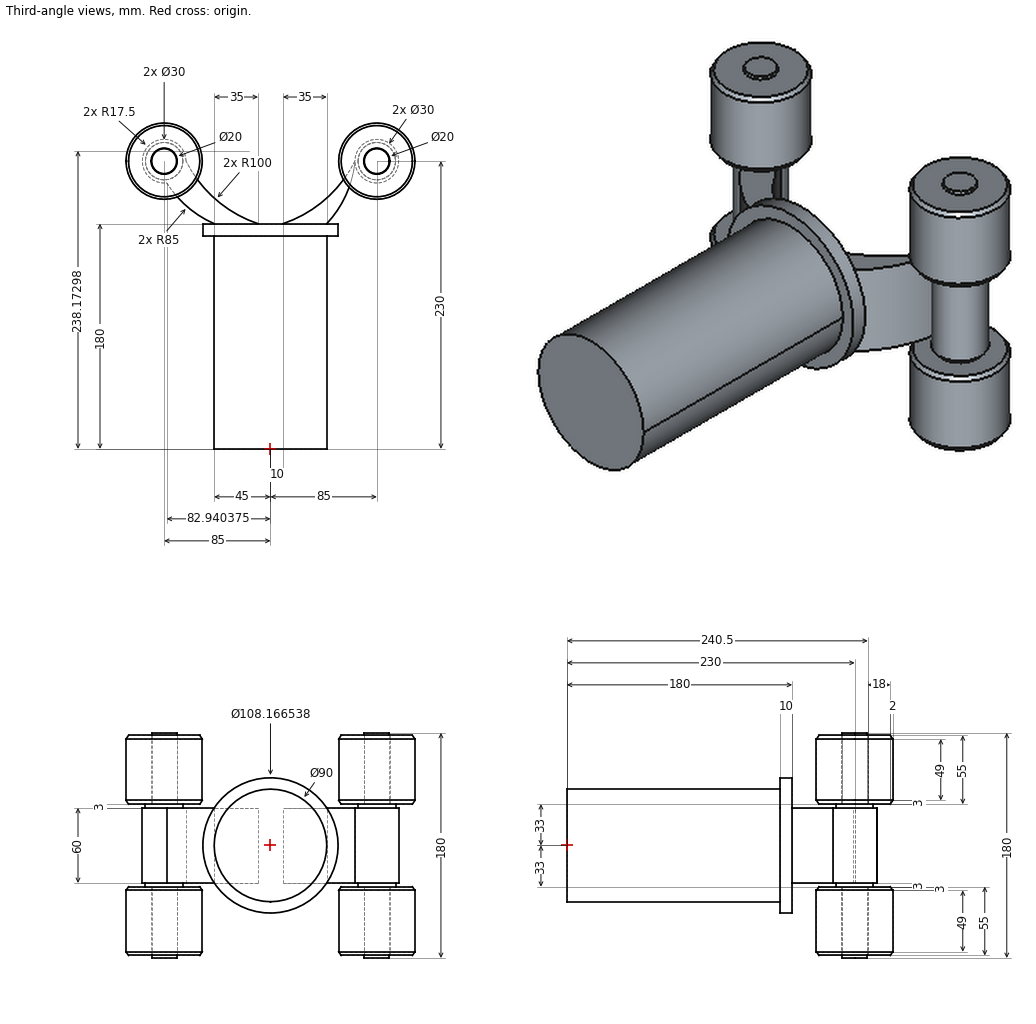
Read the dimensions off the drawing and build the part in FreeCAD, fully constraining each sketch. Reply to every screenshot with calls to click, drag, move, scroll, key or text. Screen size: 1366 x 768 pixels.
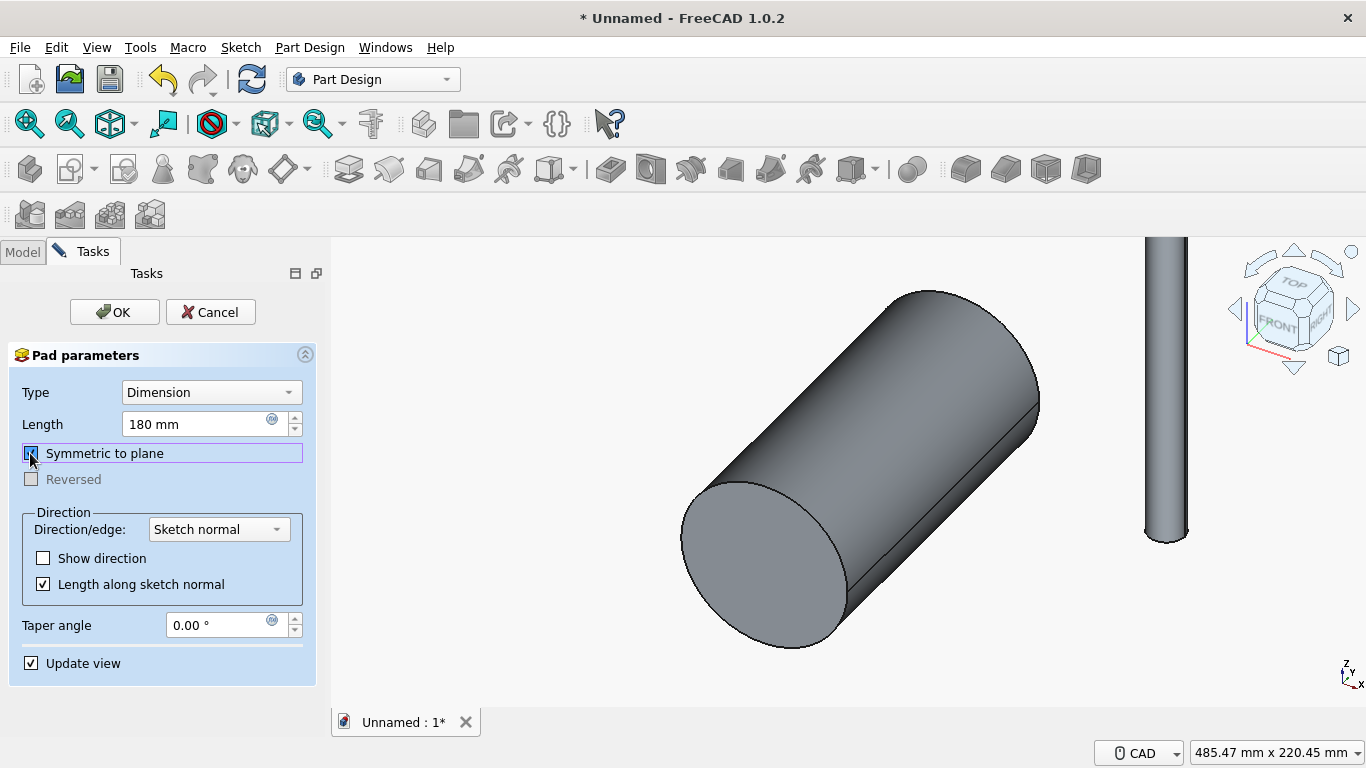
click(115, 312)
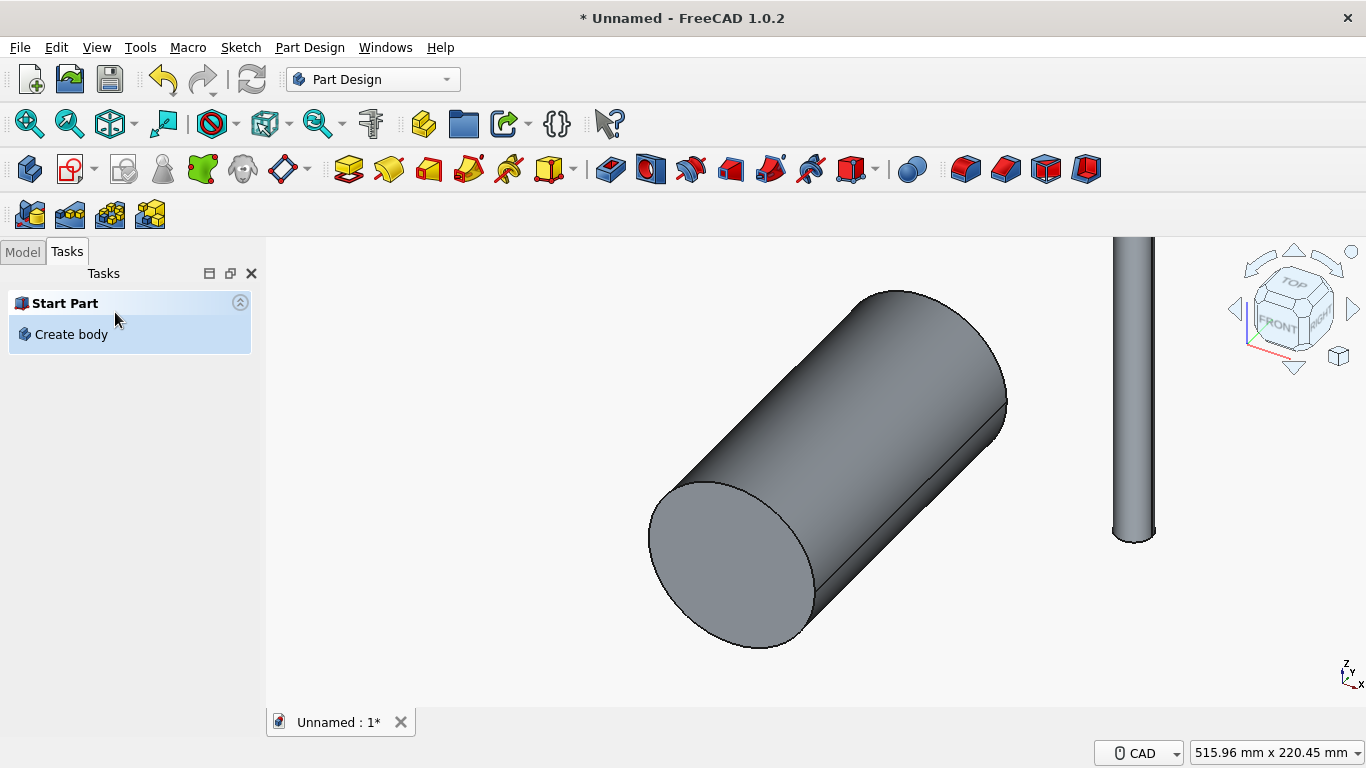
click(30, 124)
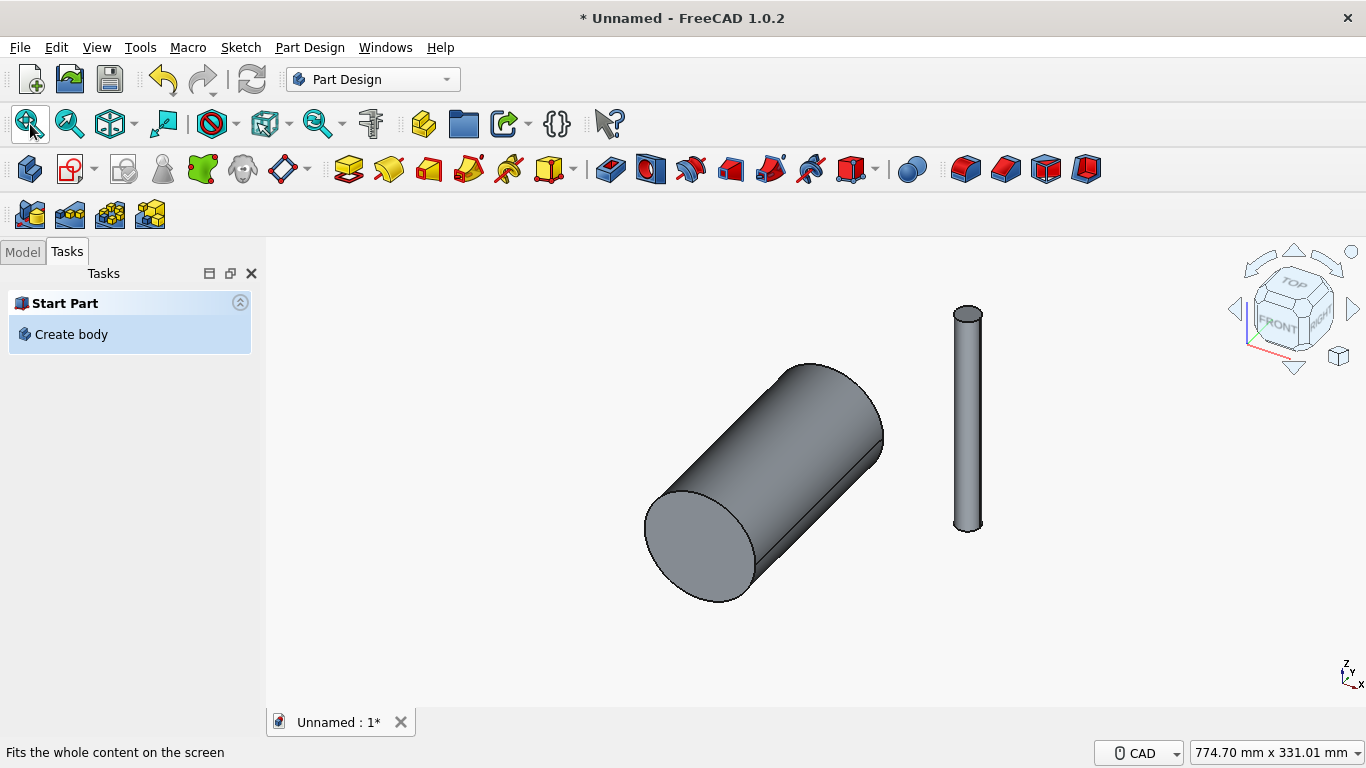
click(30, 170)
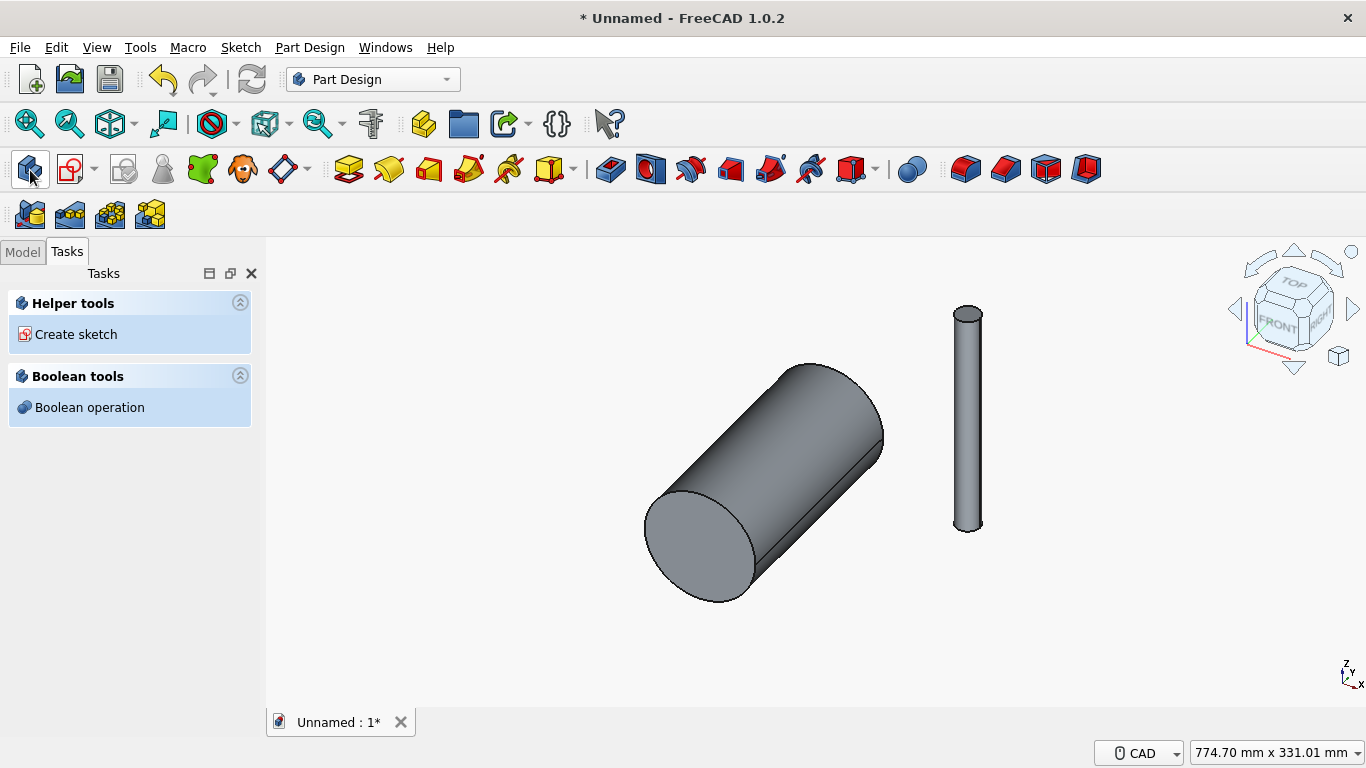
click(306, 667)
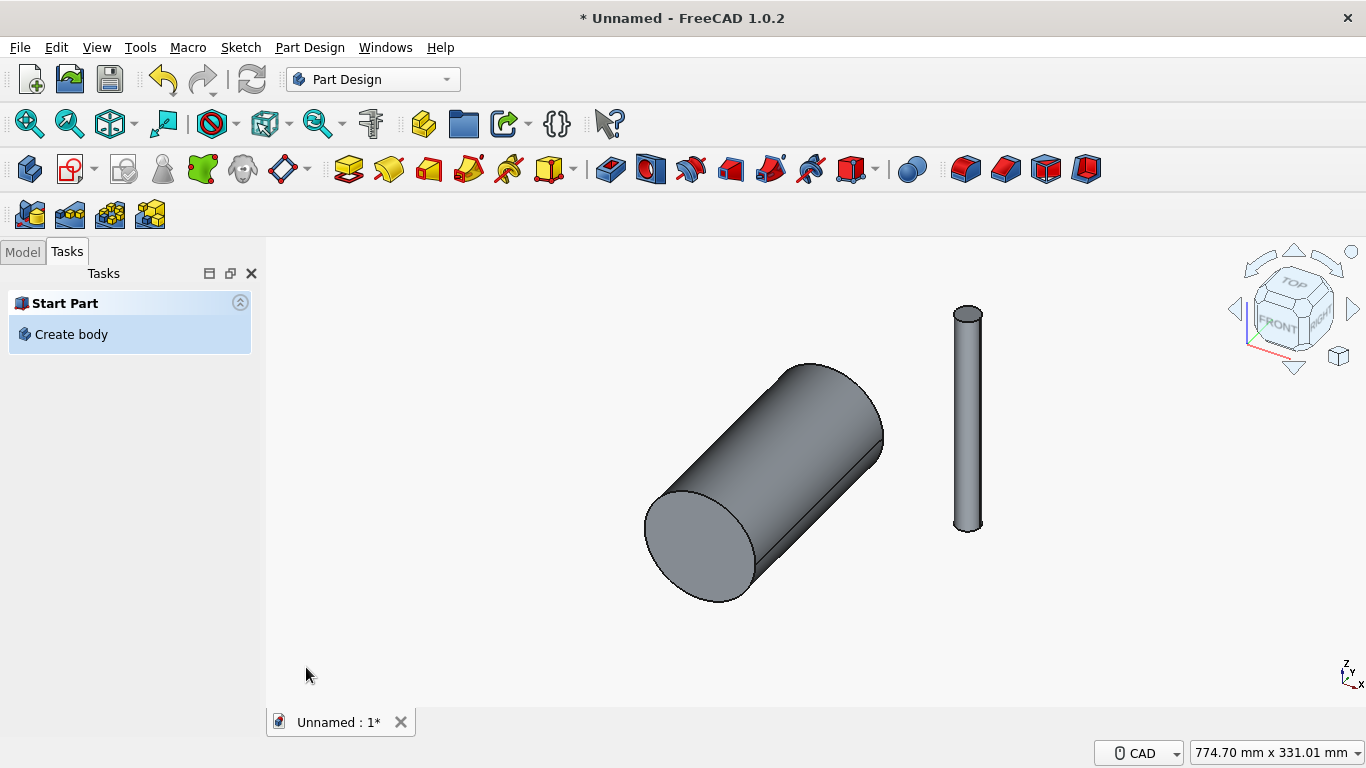
click(70, 170)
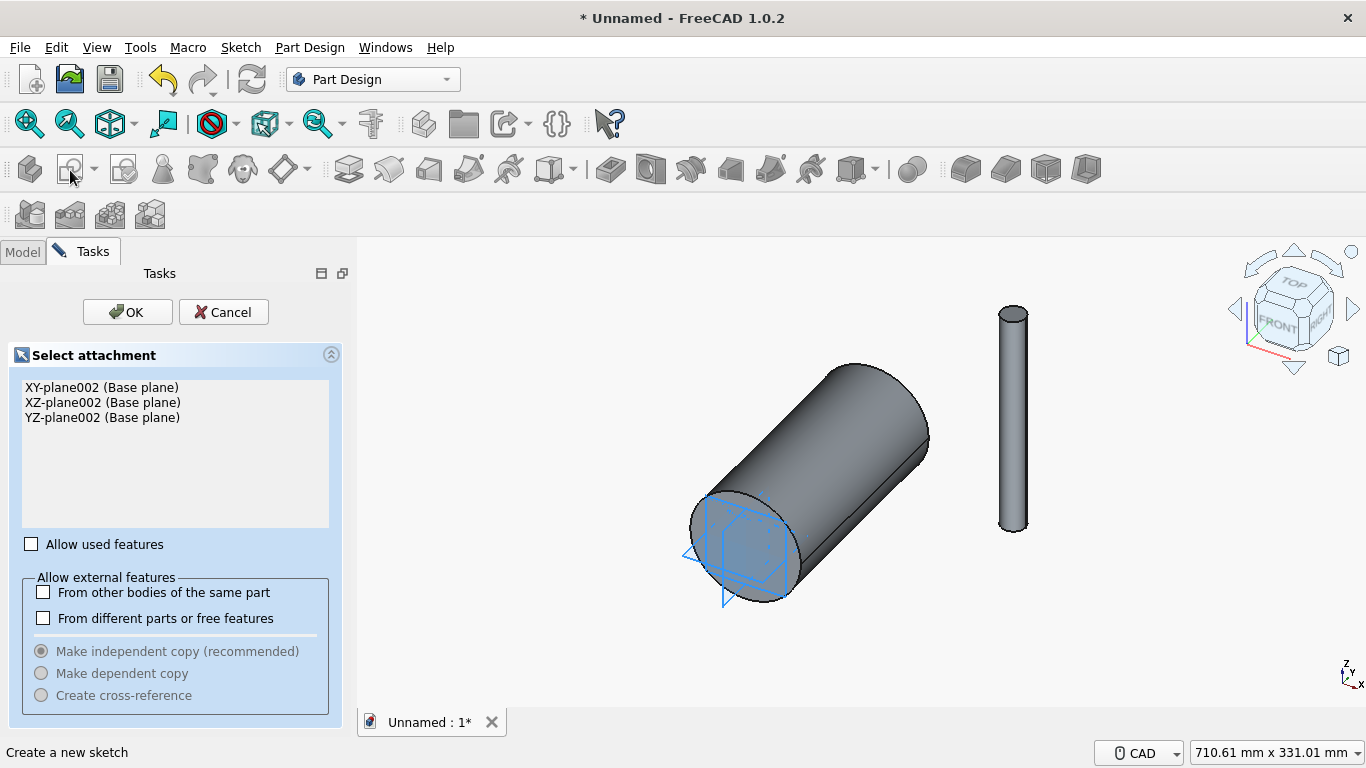
click(82, 388)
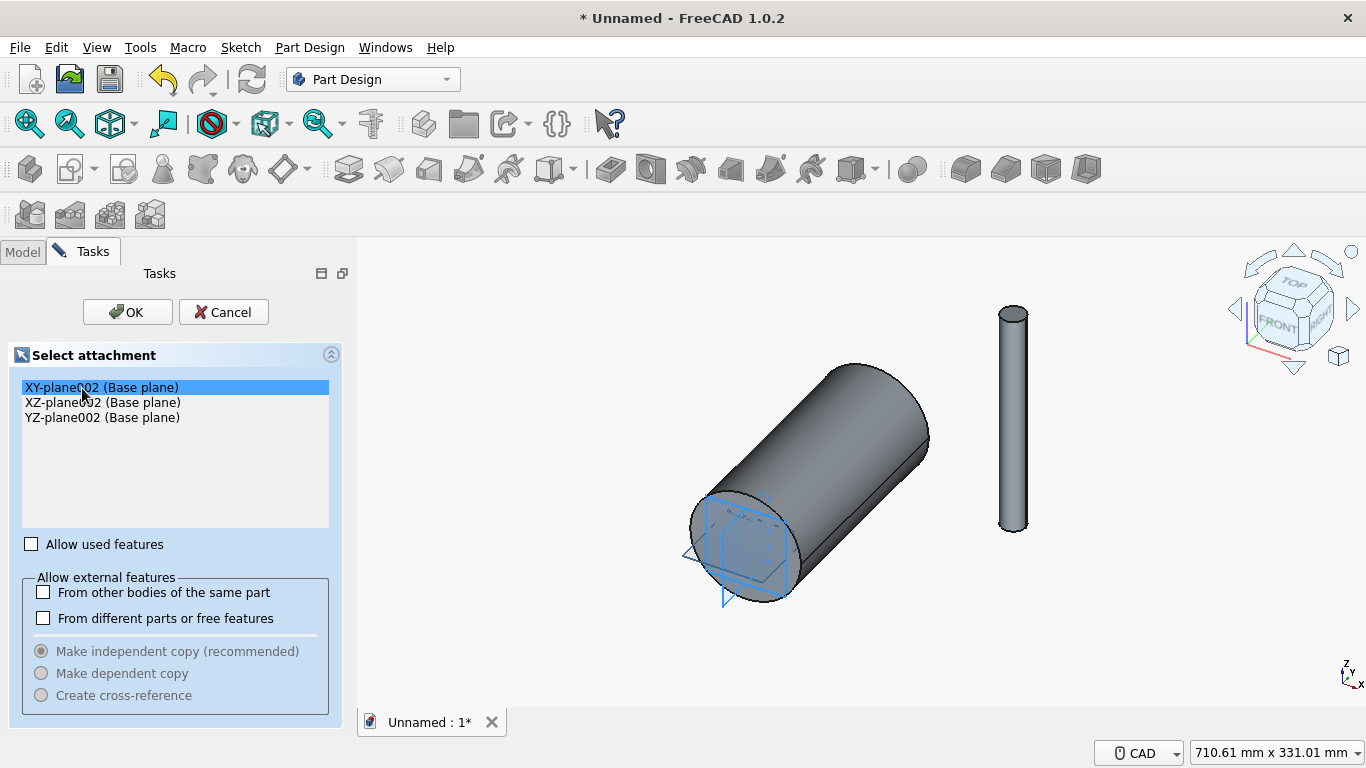
click(128, 312)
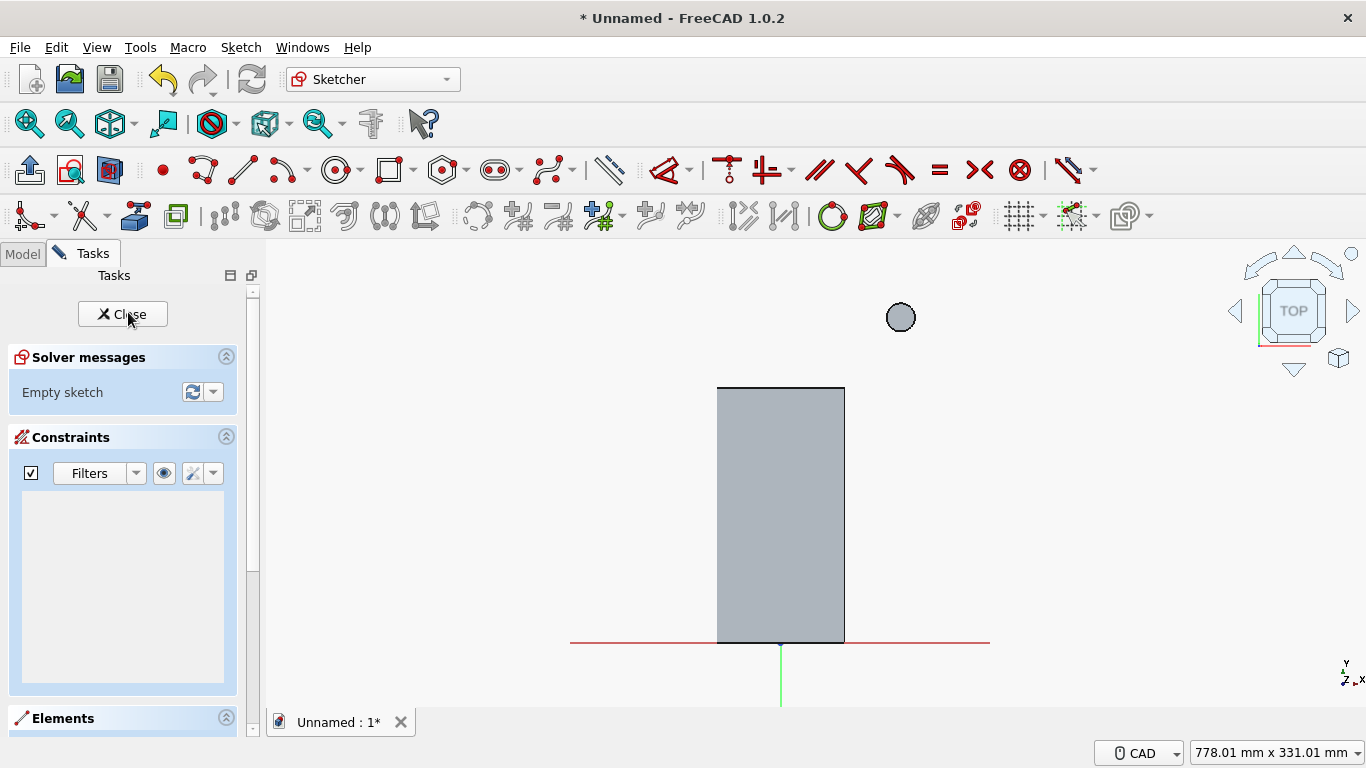
scroll(652, 302, up, 12)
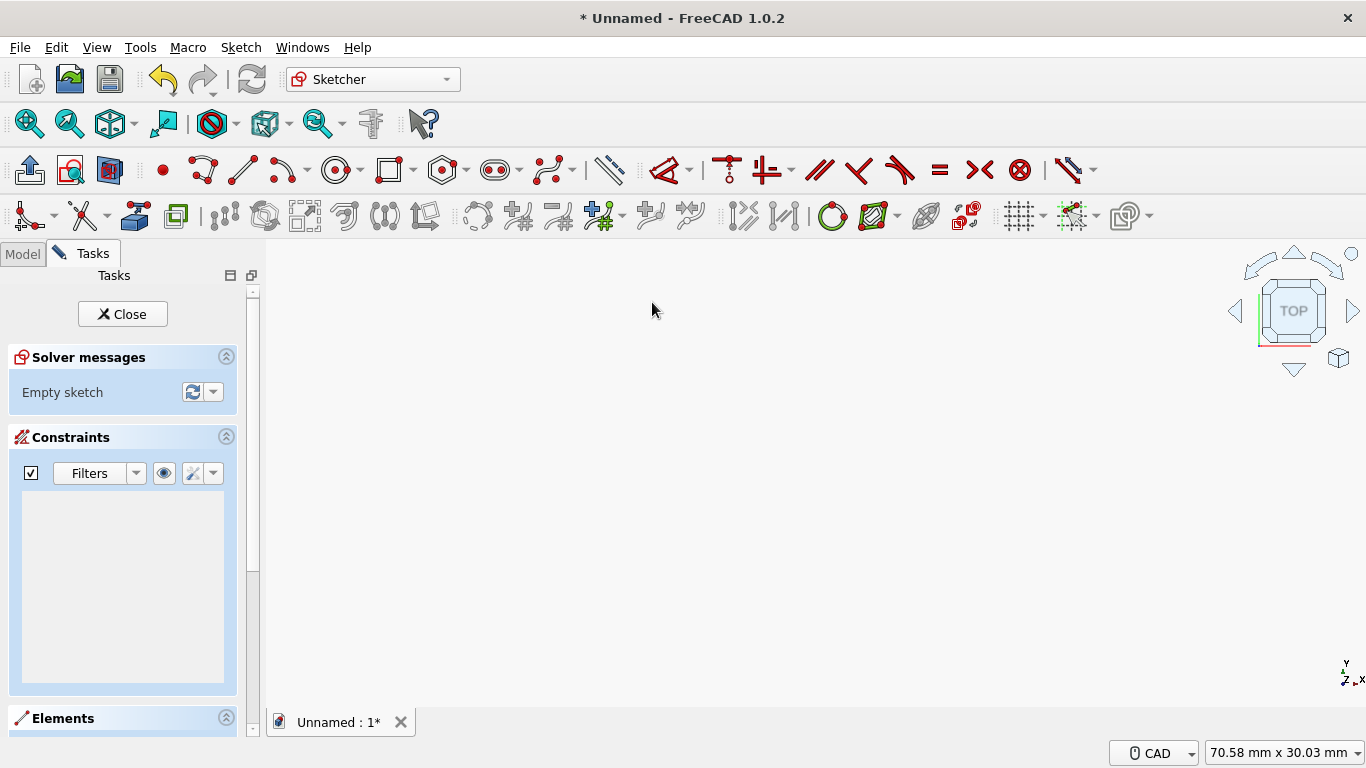
click(336, 170)